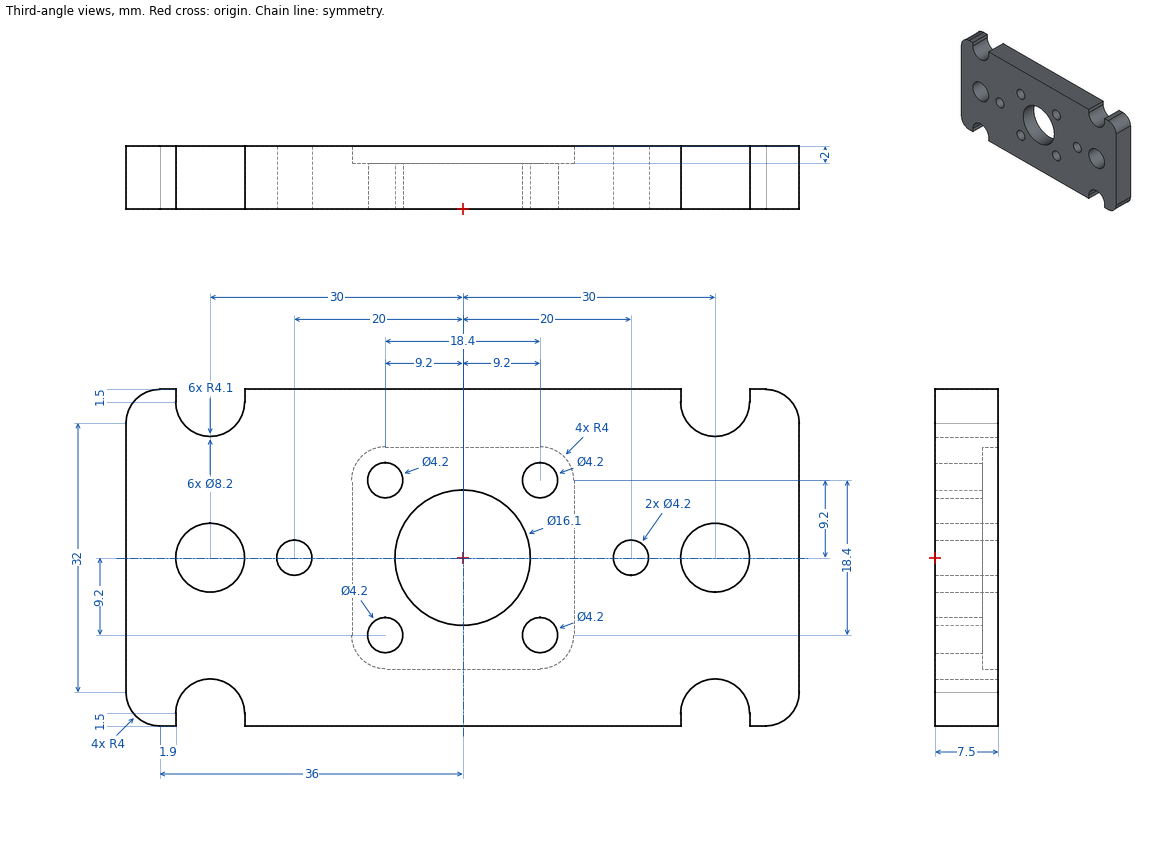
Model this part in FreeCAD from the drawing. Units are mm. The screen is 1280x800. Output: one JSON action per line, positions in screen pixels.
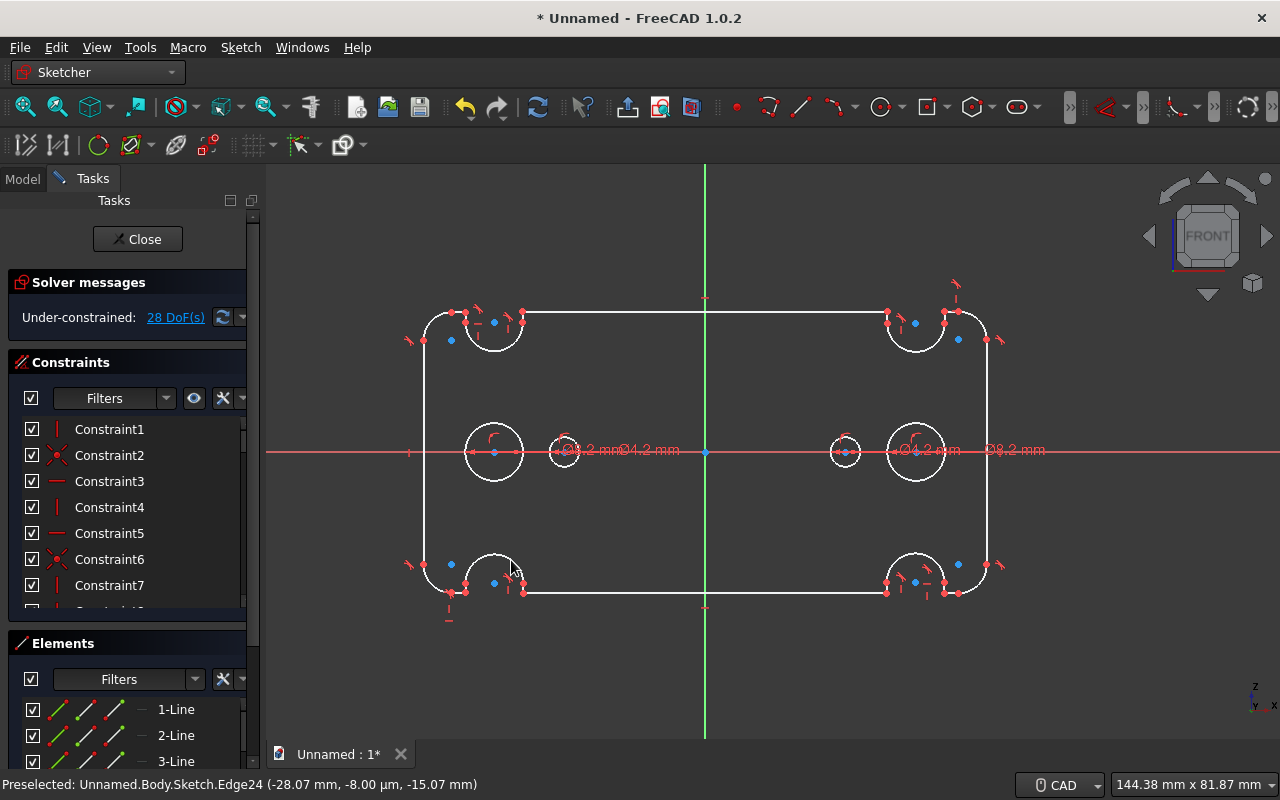
{"action": "left_click", "coordinate": [427, 578]}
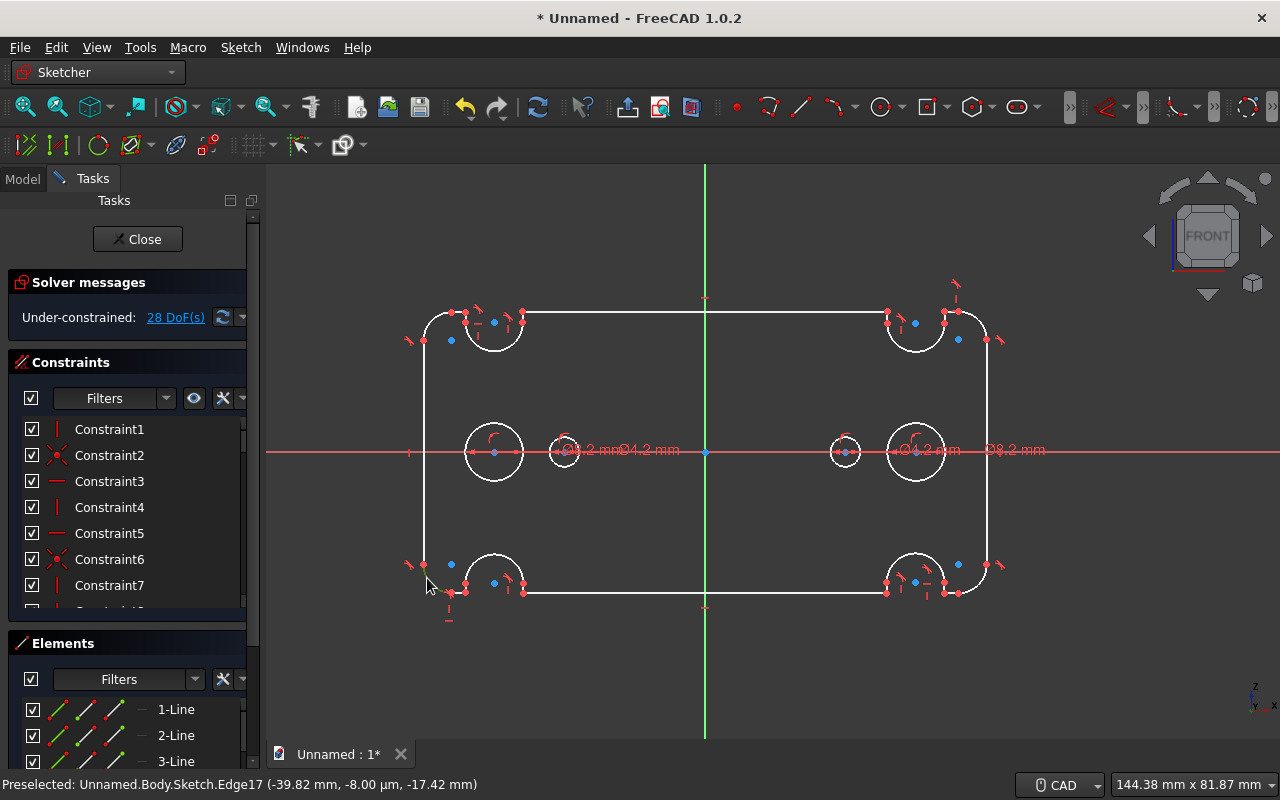
{"action": "left_click", "coordinate": [439, 315]}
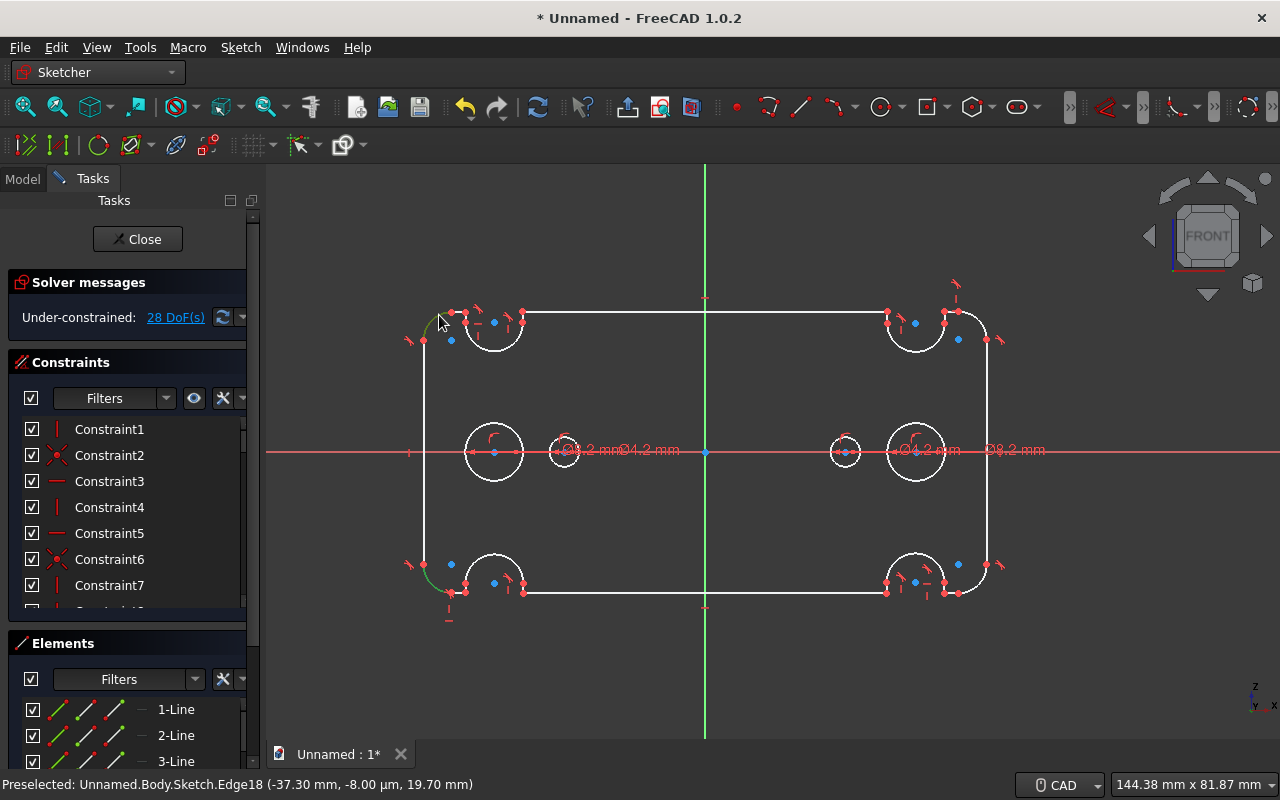
{"action": "left_click", "coordinate": [984, 327]}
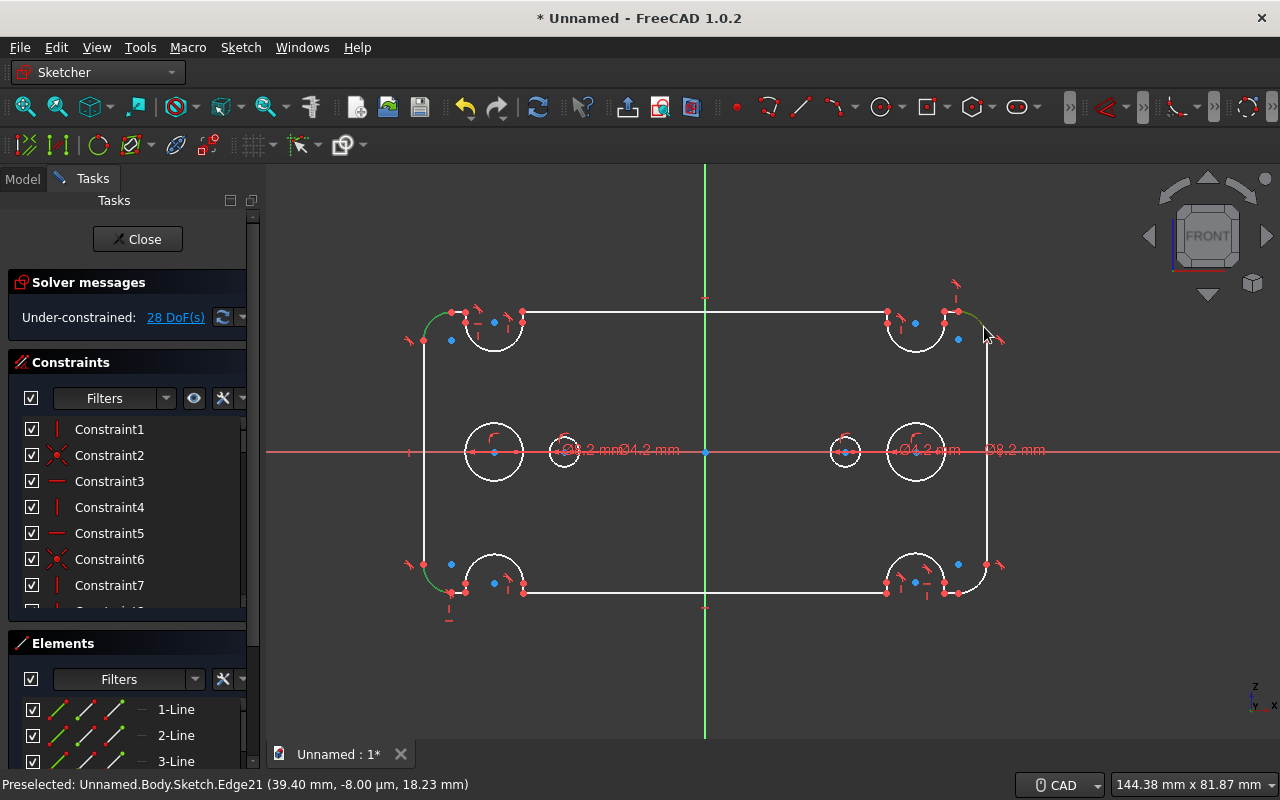
{"action": "left_click", "coordinate": [971, 590]}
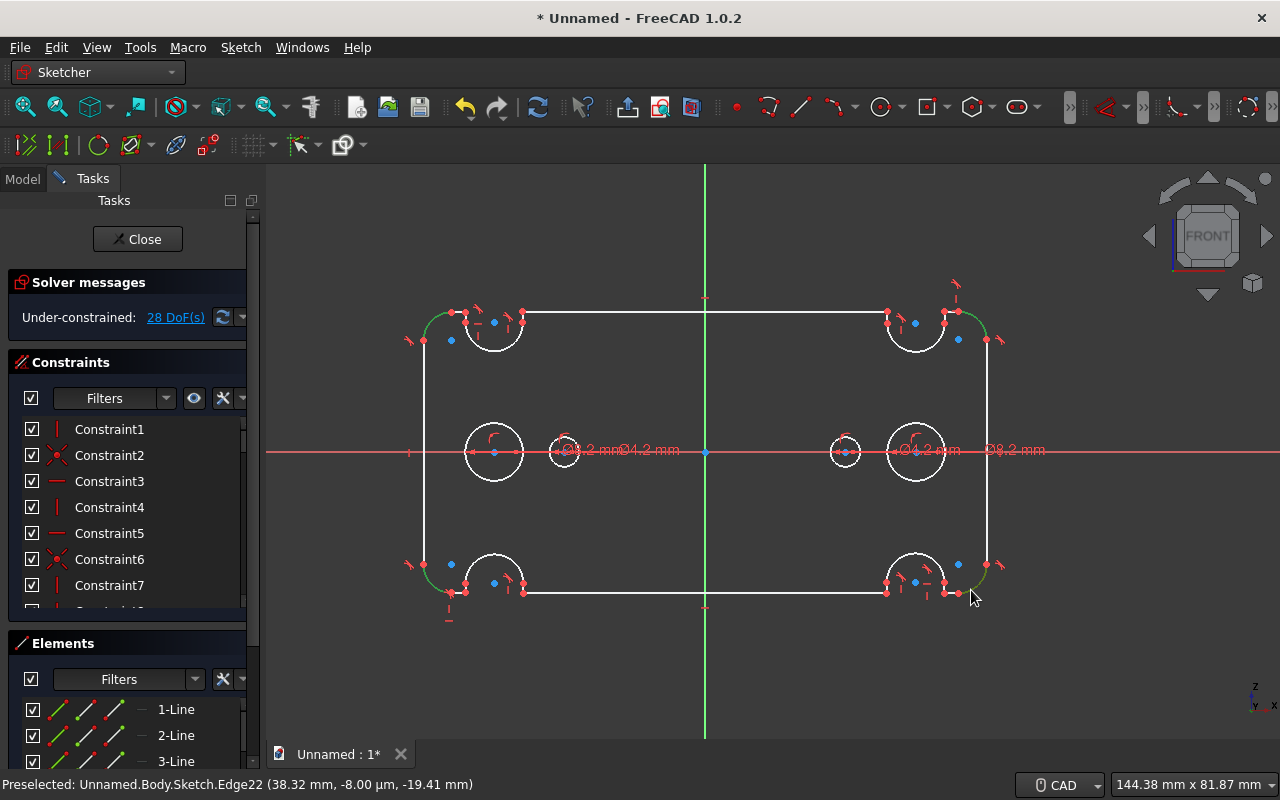
{"action": "key", "text": "e"}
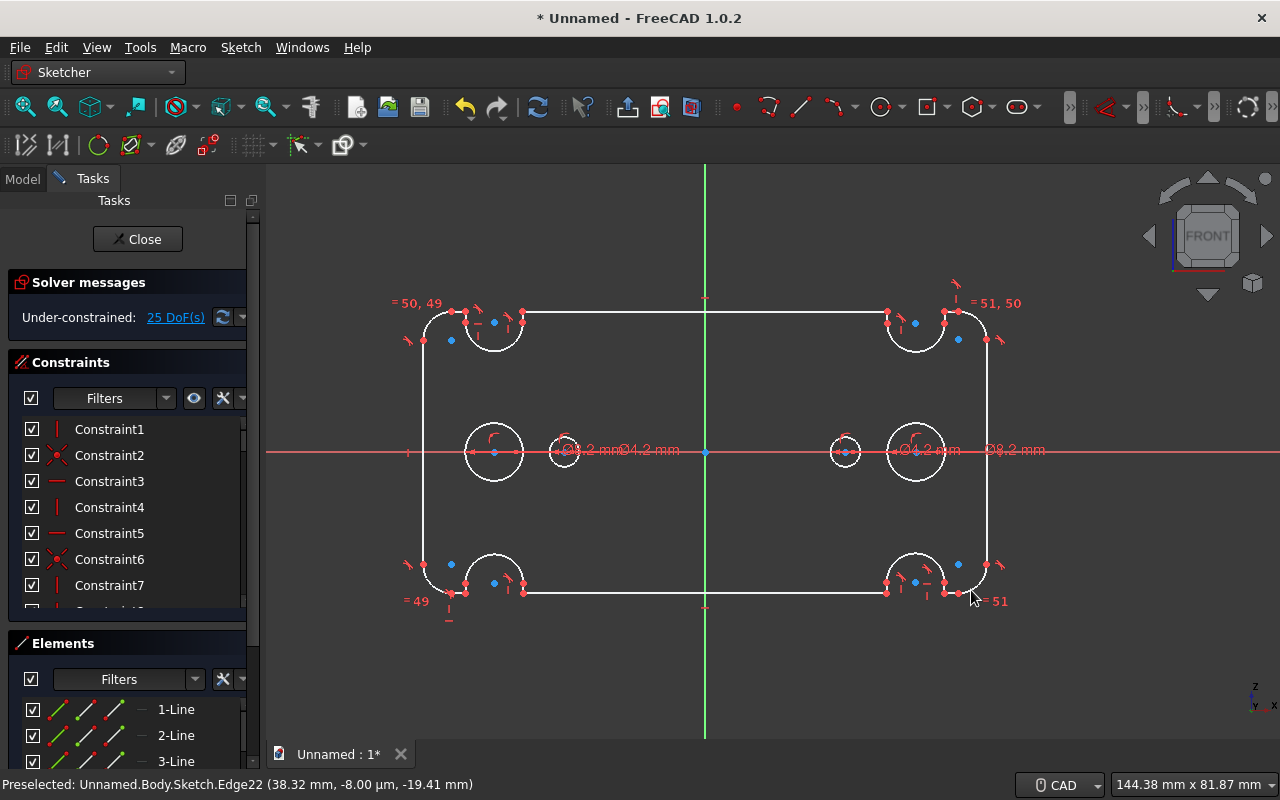
{"action": "left_click", "coordinate": [477, 346]}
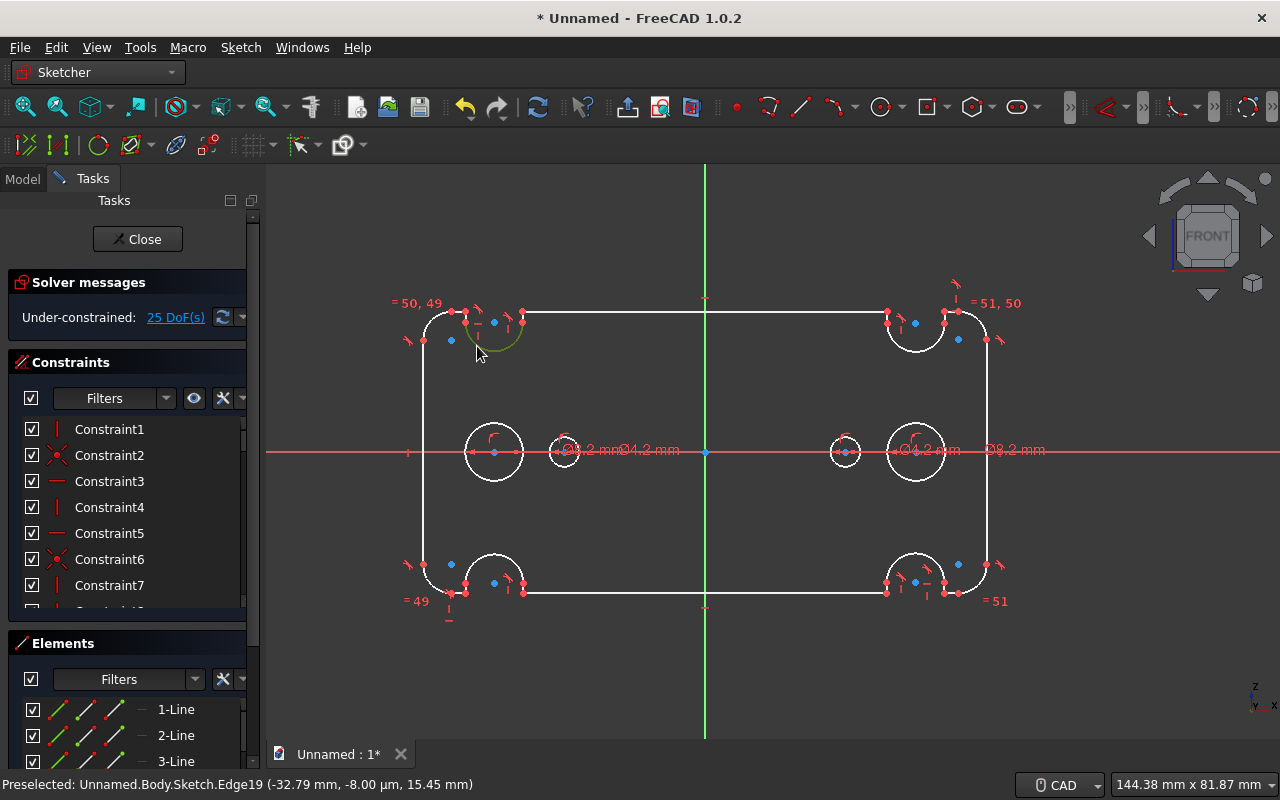
{"action": "left_click", "coordinate": [899, 346]}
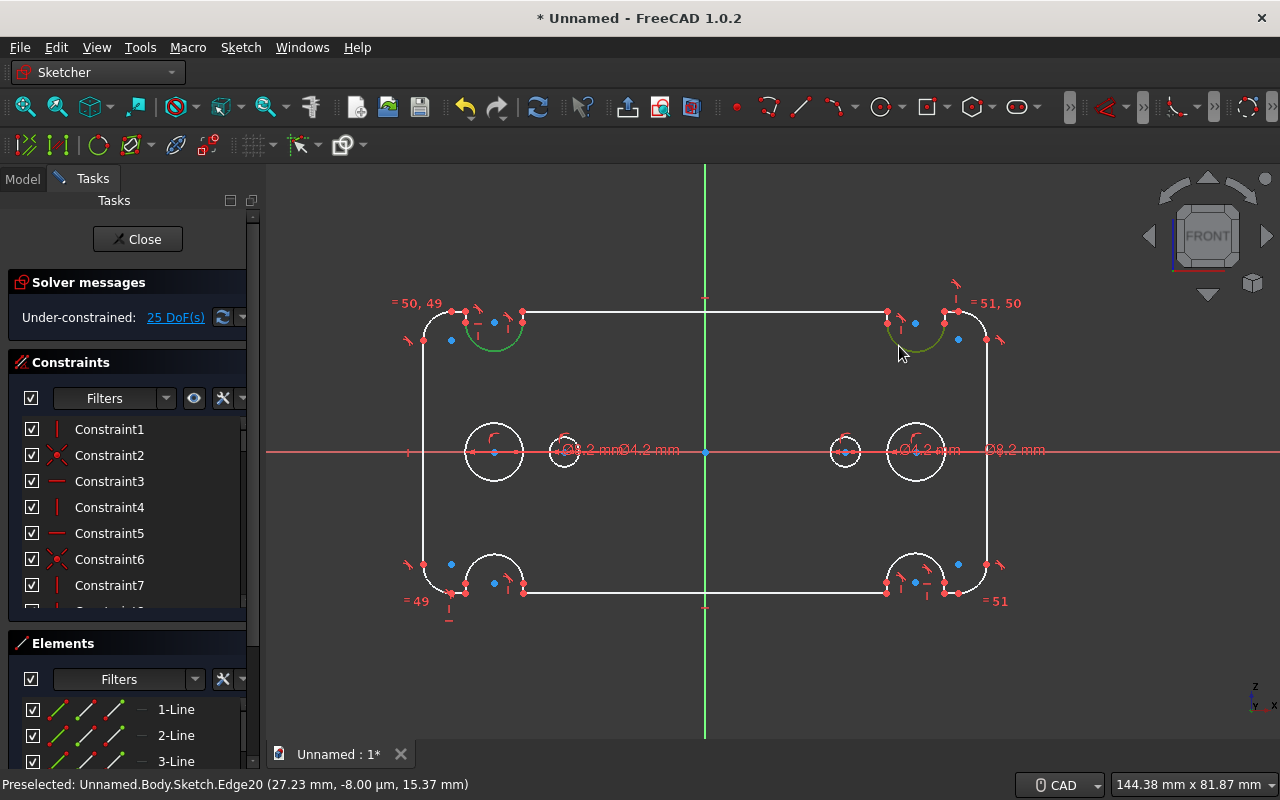
{"action": "left_click", "coordinate": [932, 559]}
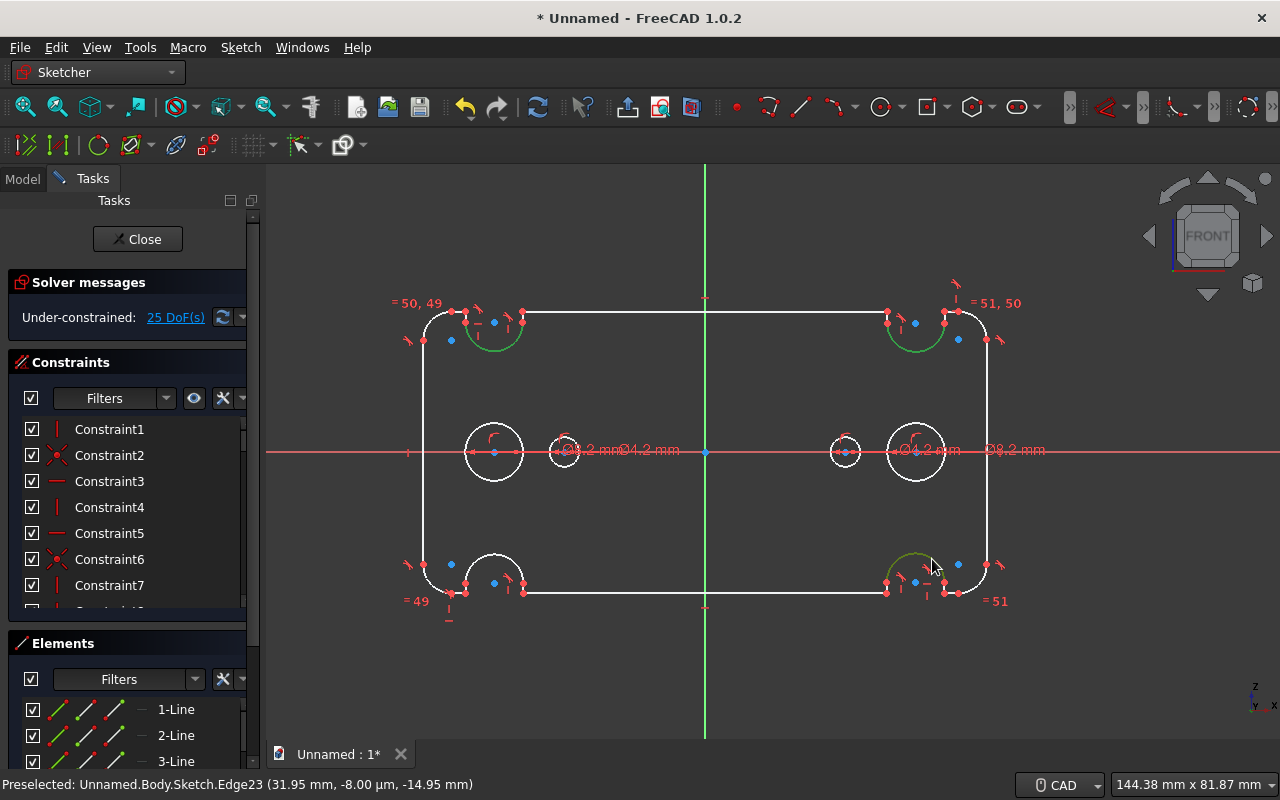
{"action": "left_click", "coordinate": [511, 560]}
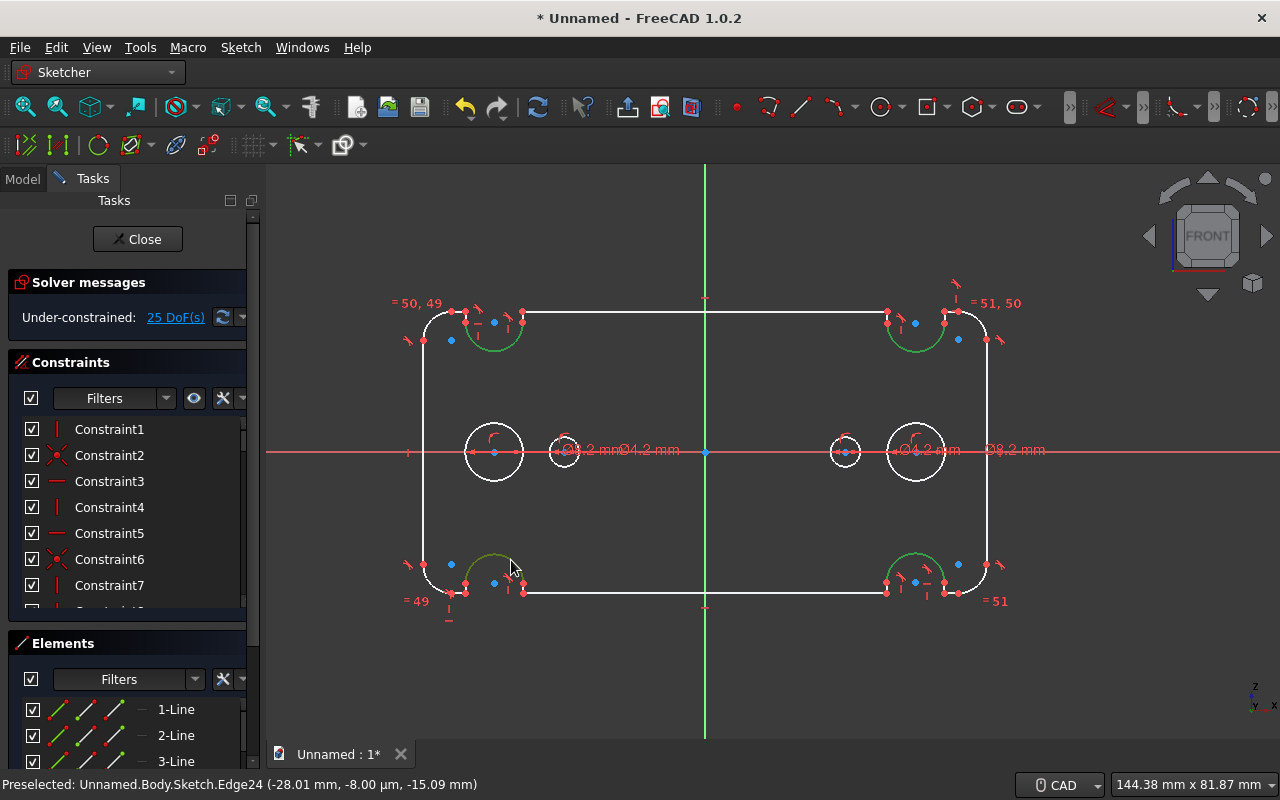
{"action": "key", "text": "e"}